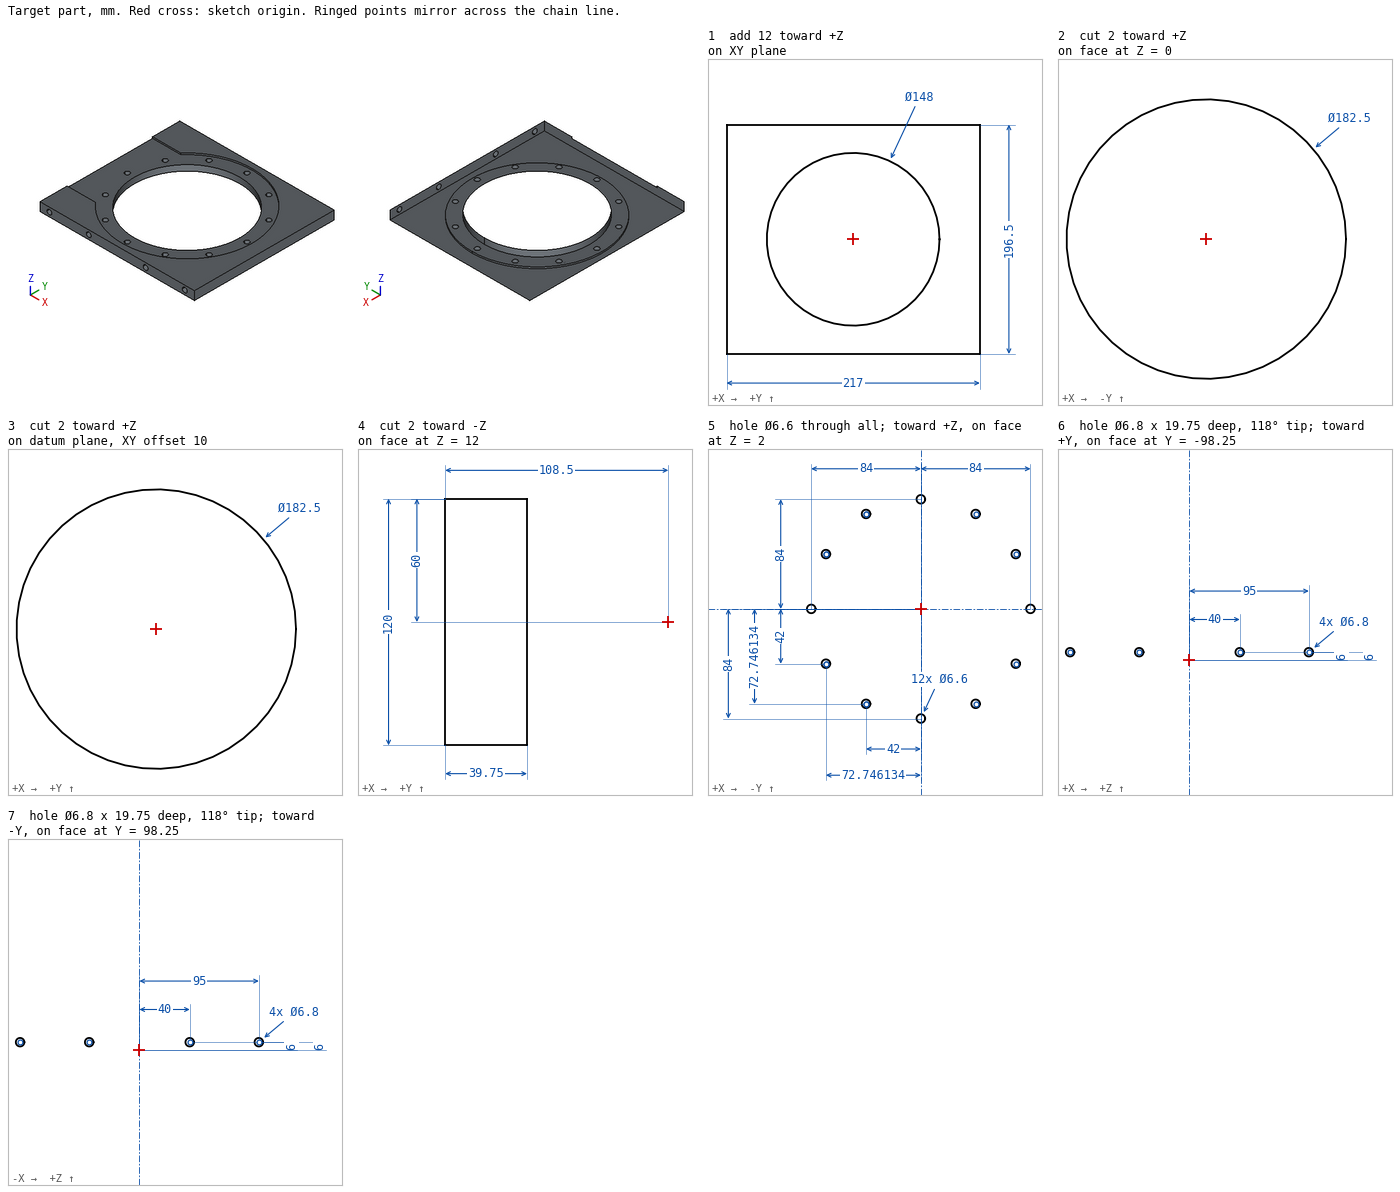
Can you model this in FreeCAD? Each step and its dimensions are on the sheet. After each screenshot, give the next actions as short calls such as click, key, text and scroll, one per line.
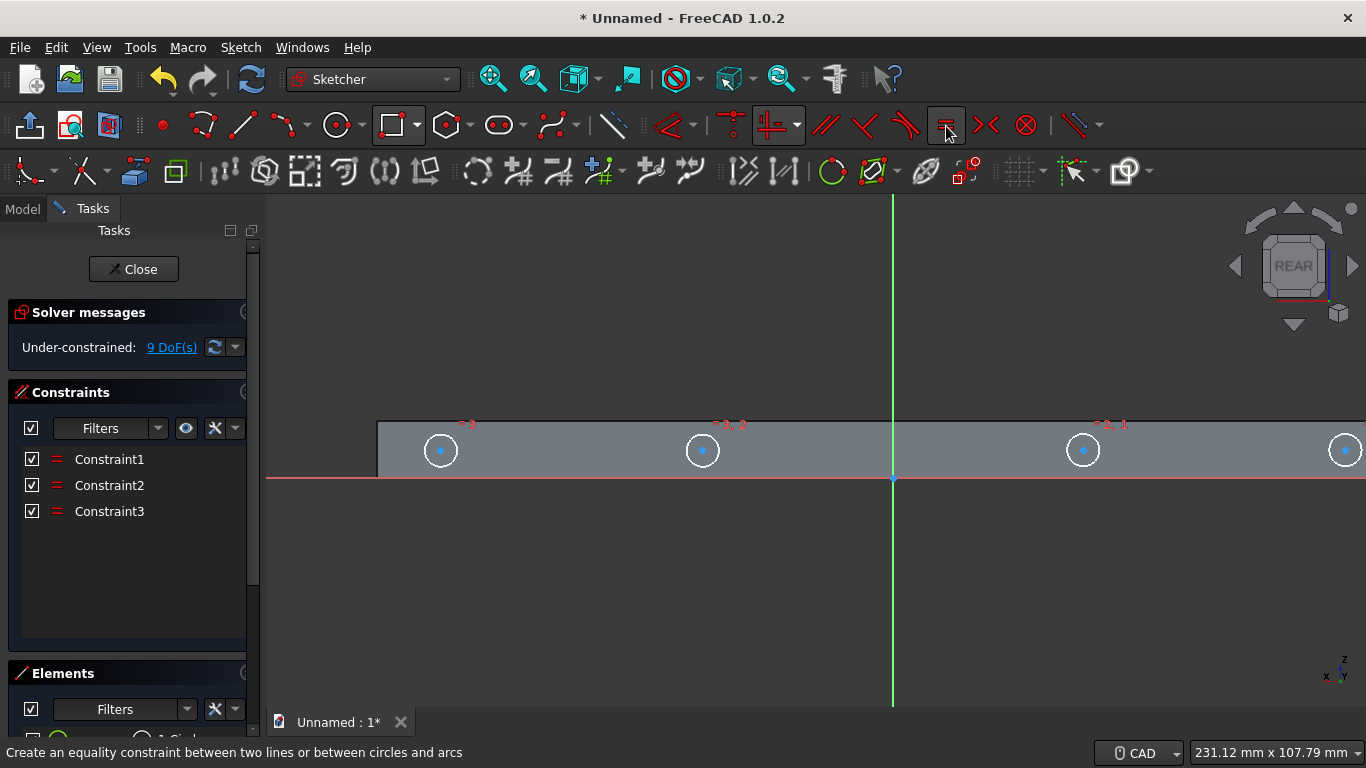
click(1083, 450)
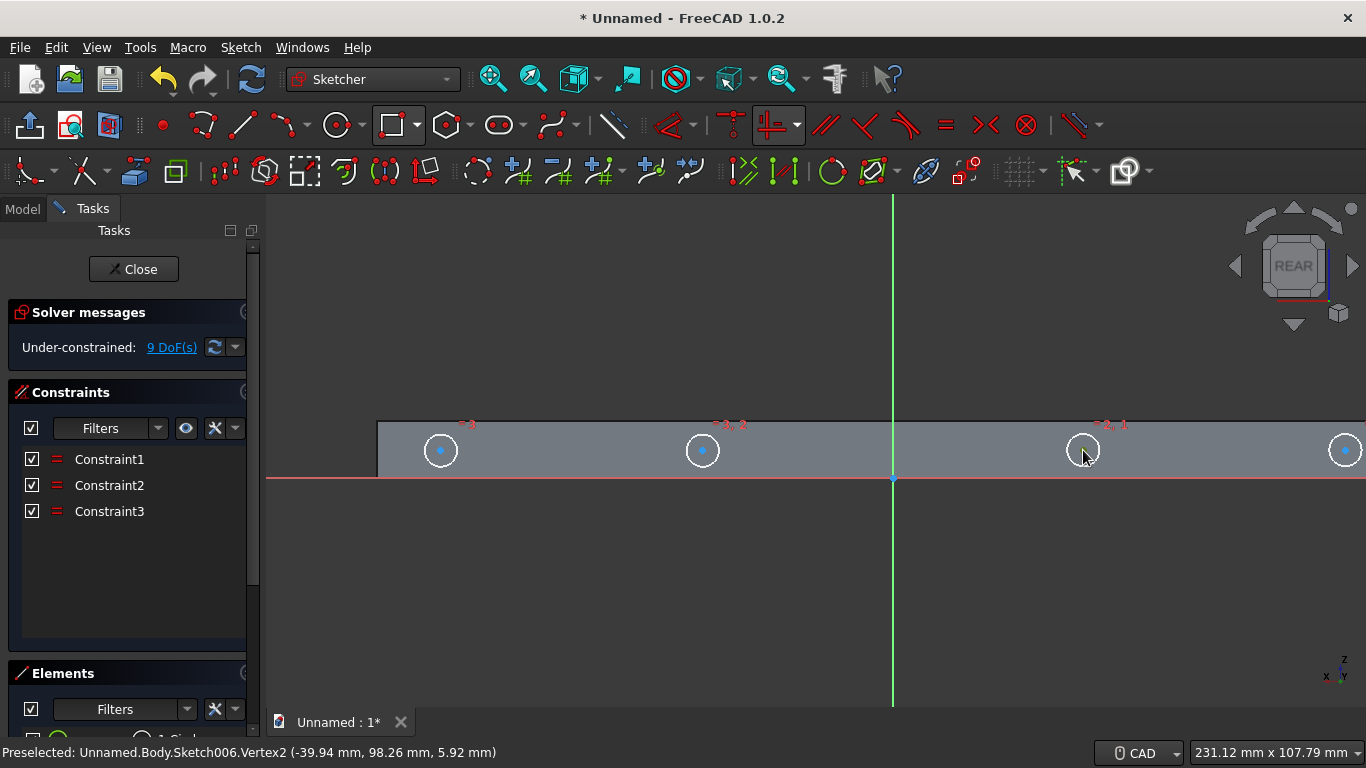
click(703, 451)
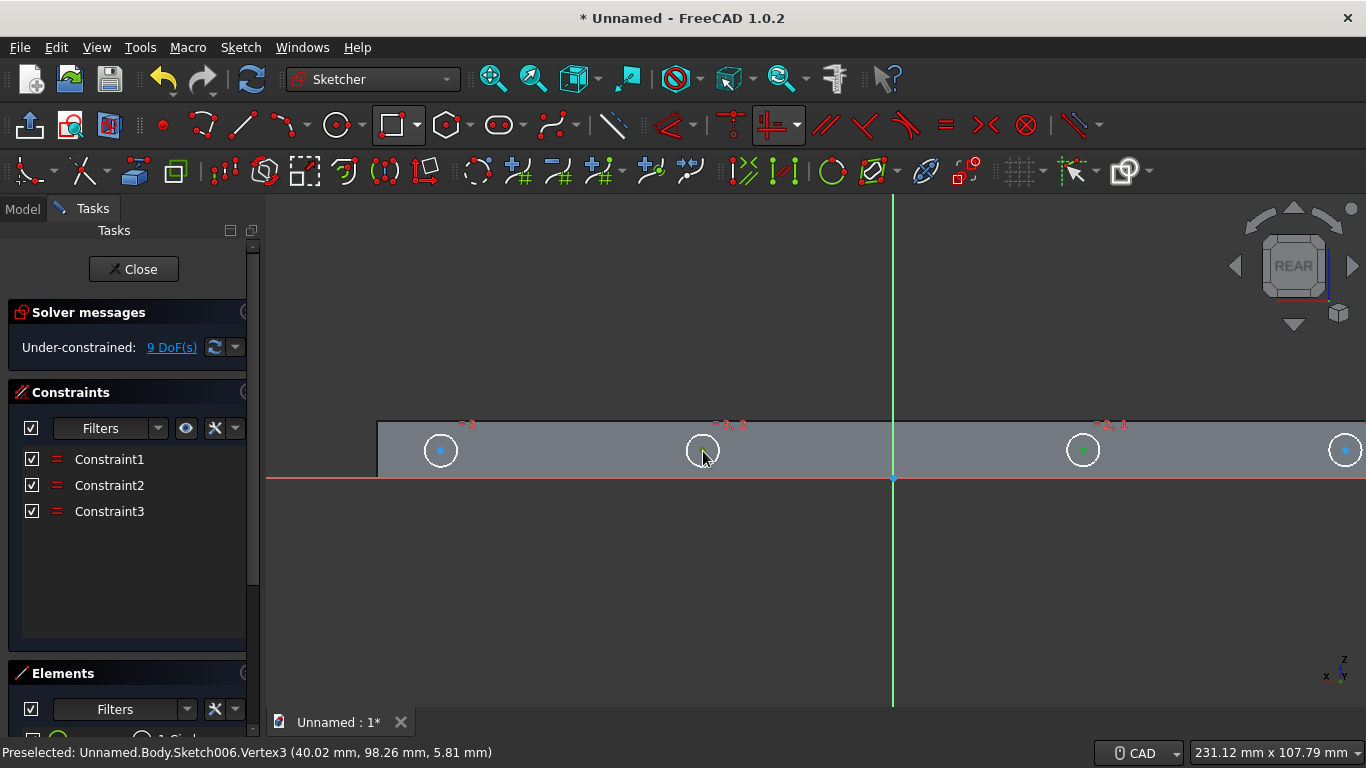
click(893, 646)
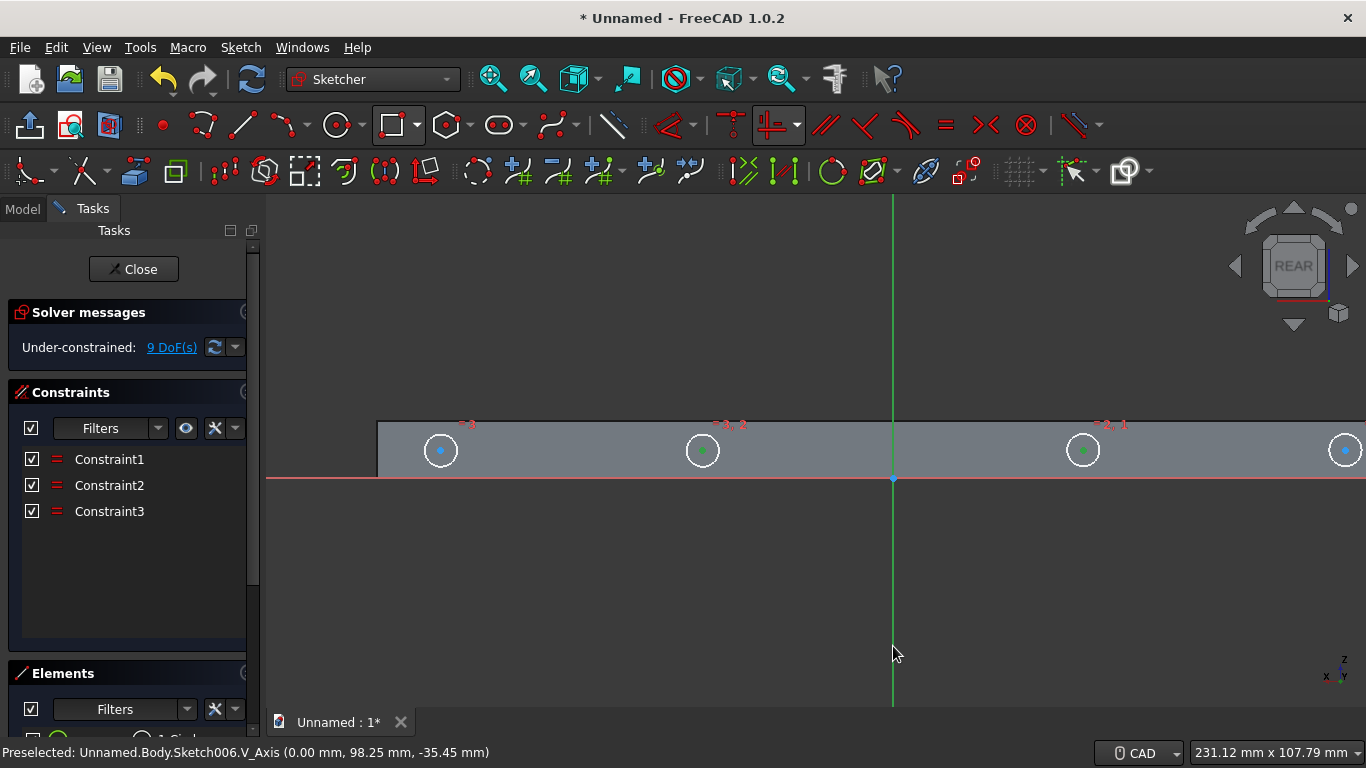
click(986, 126)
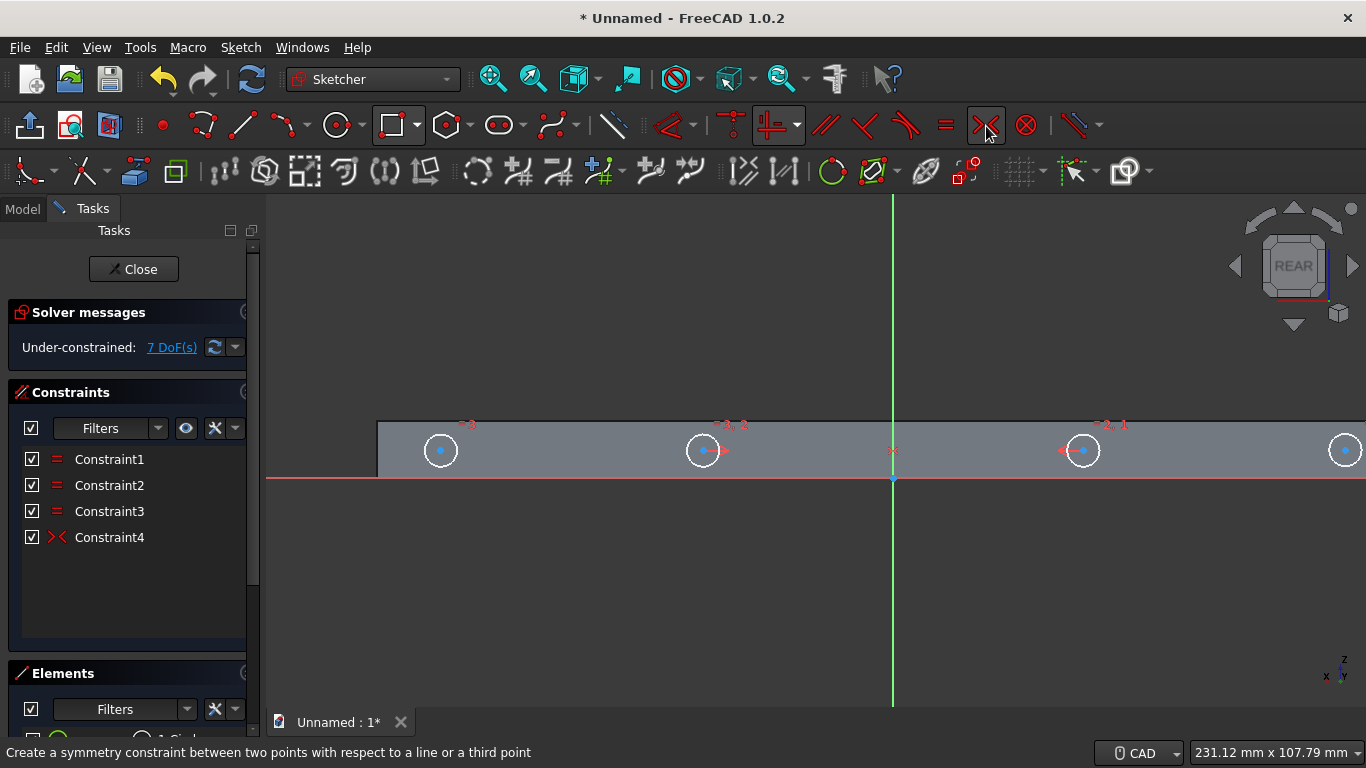
scroll(451, 440, down, 2)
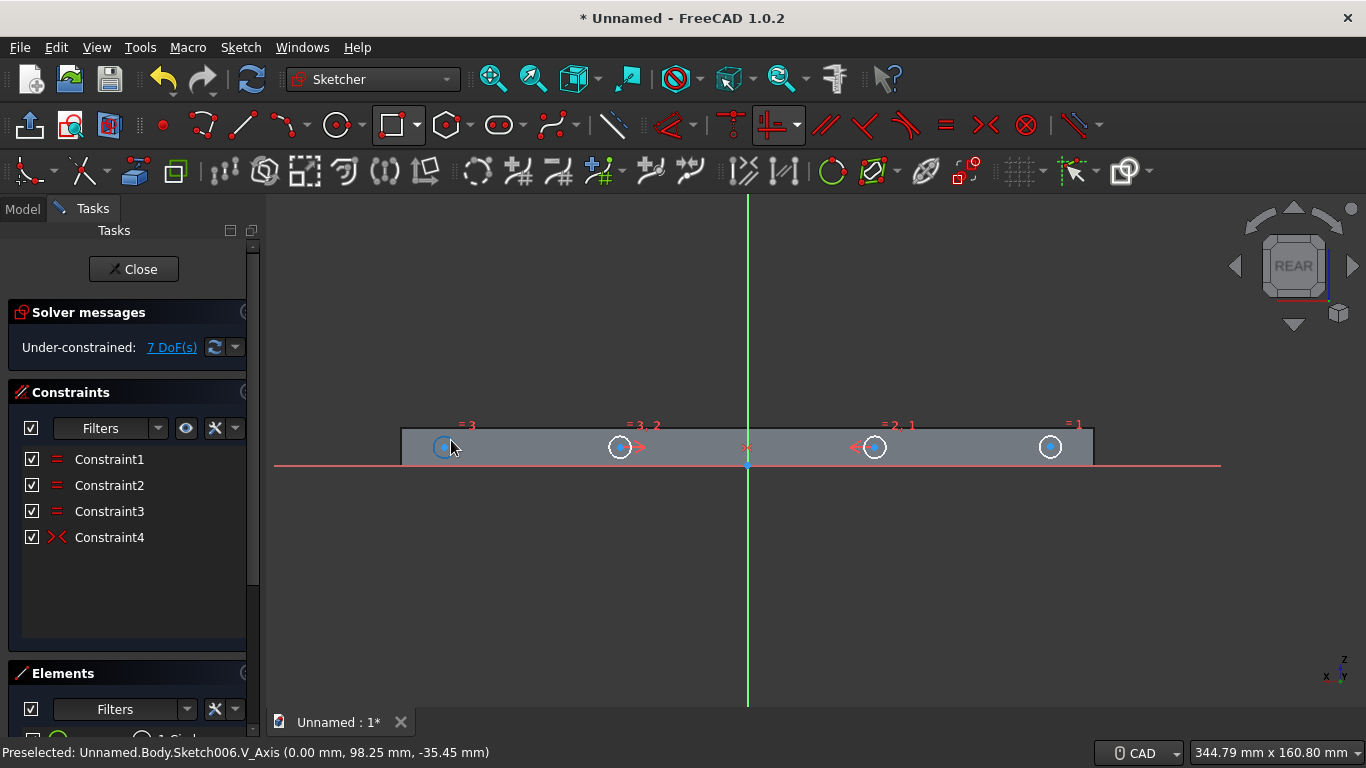
click(1051, 447)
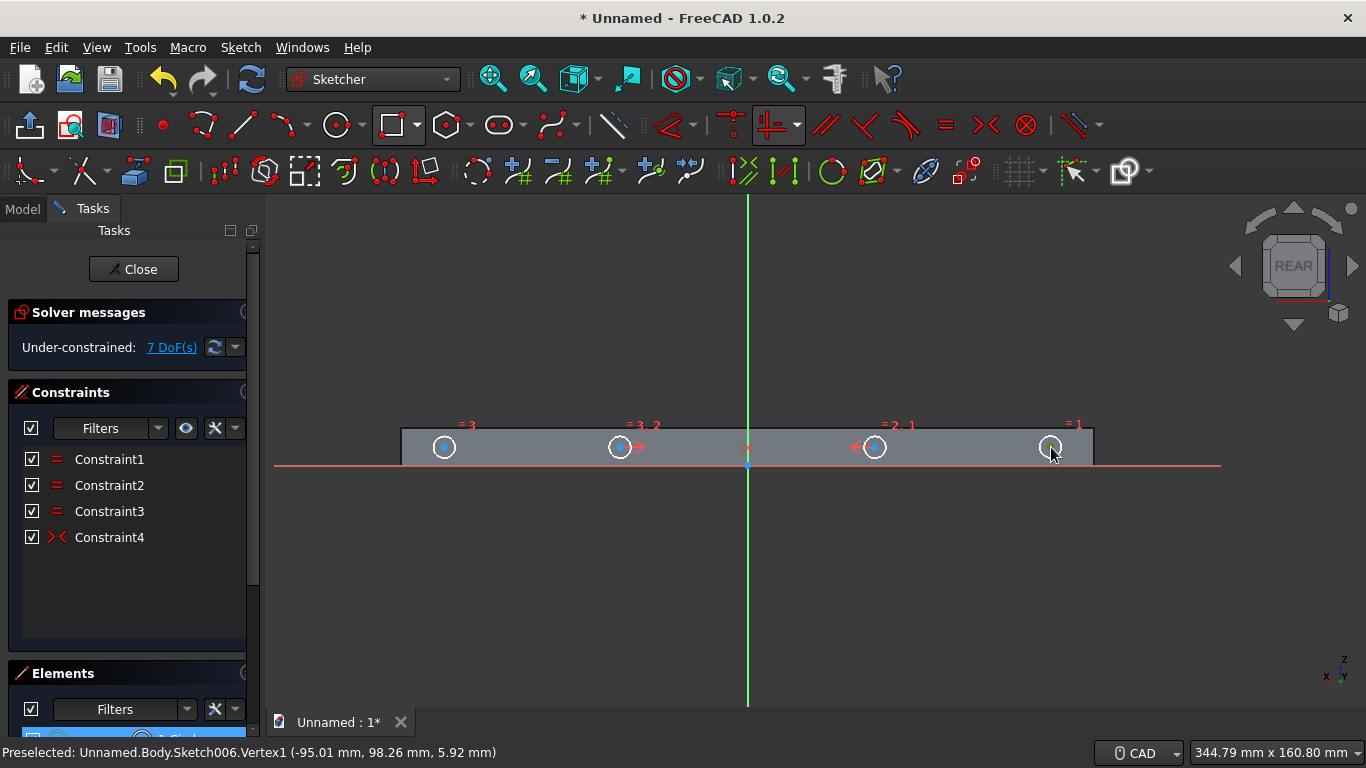
click(444, 447)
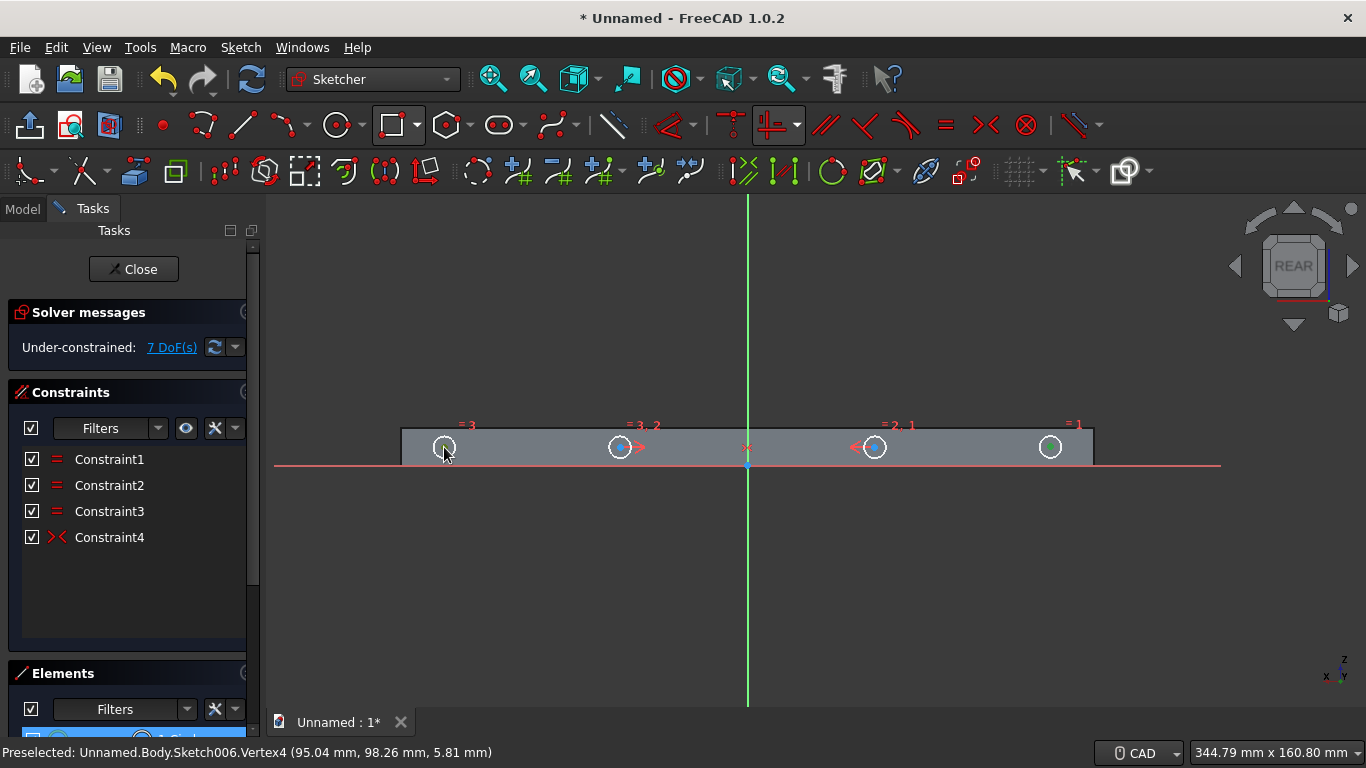
click(748, 646)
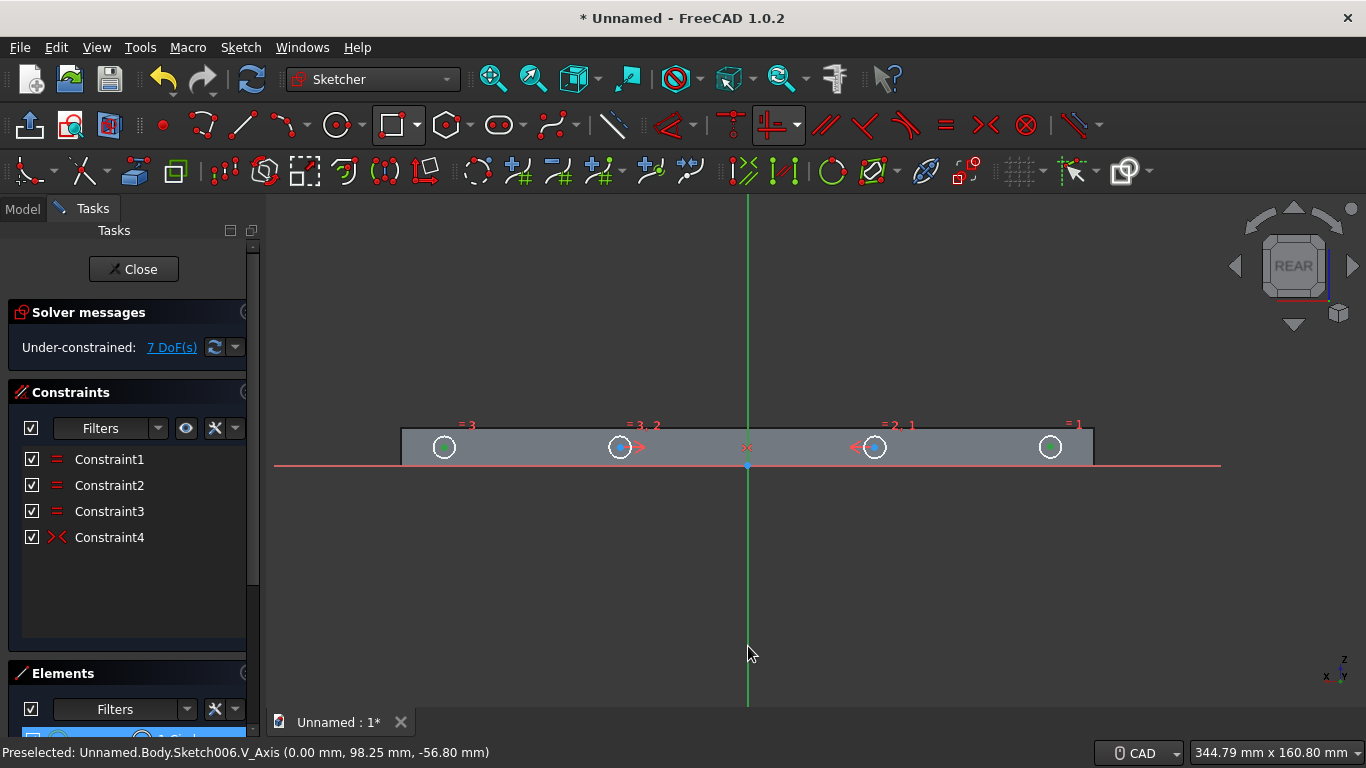
click(986, 126)